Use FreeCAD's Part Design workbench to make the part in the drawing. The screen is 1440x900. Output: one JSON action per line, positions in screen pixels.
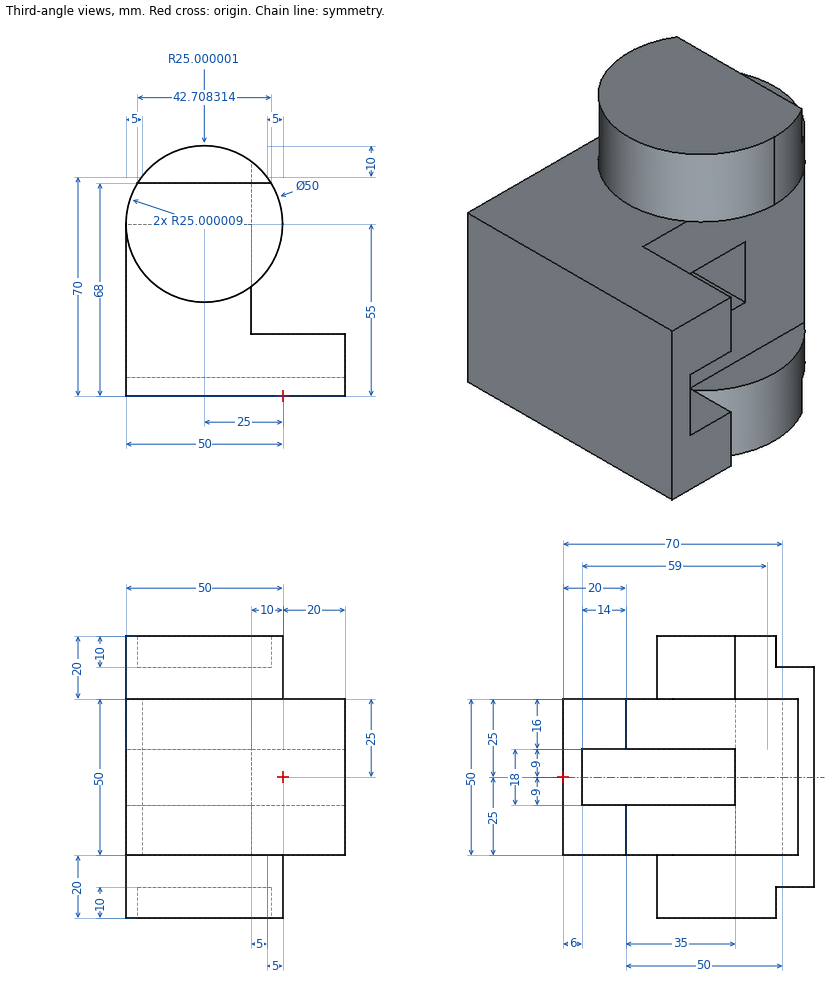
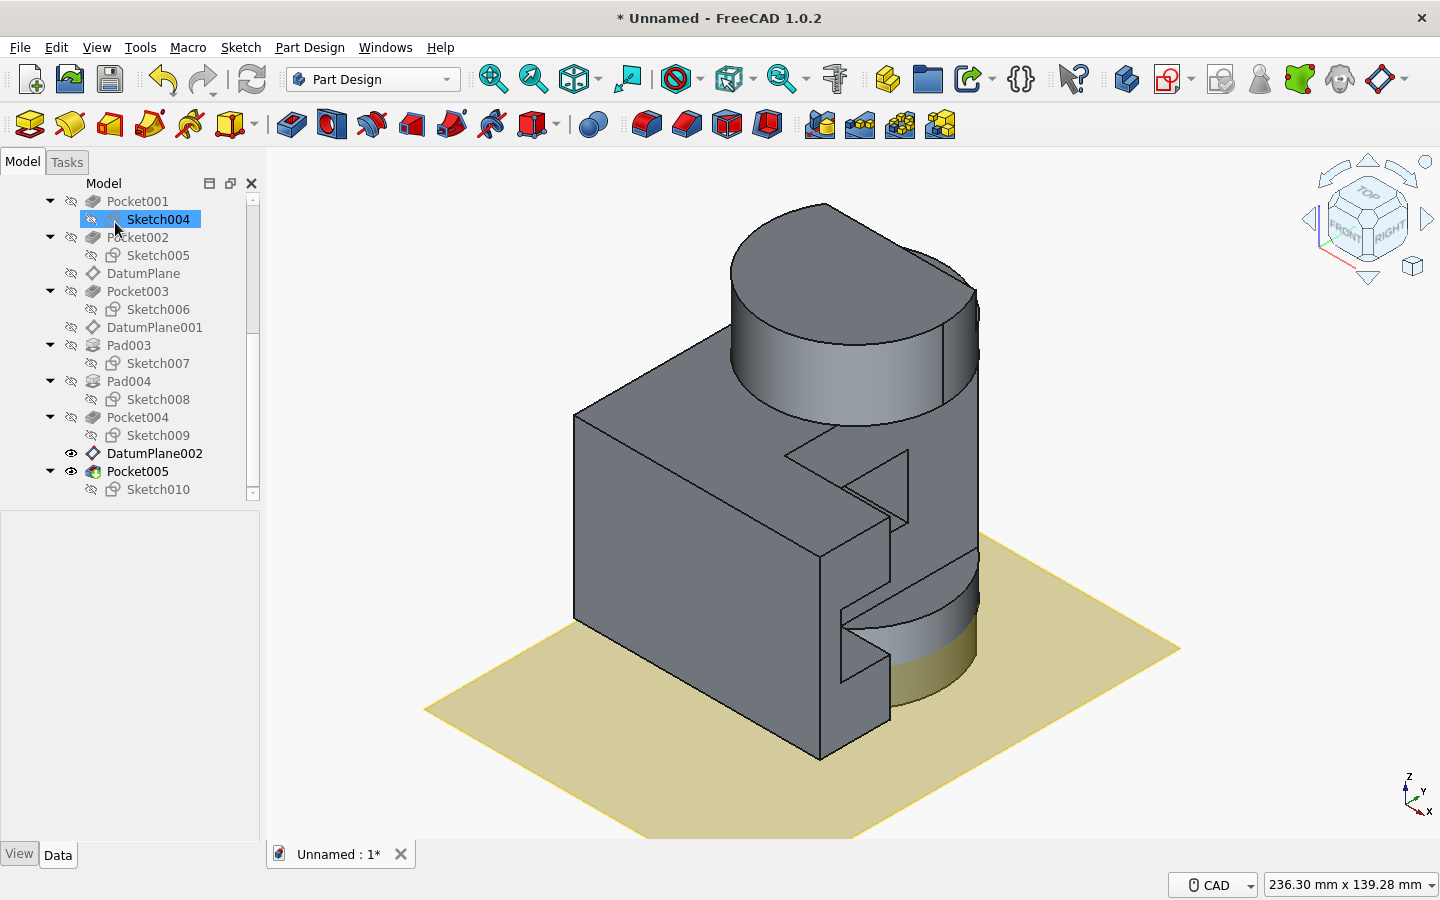
{"action": "left_click", "coordinate": [116, 453]}
{"action": "key", "text": "space"}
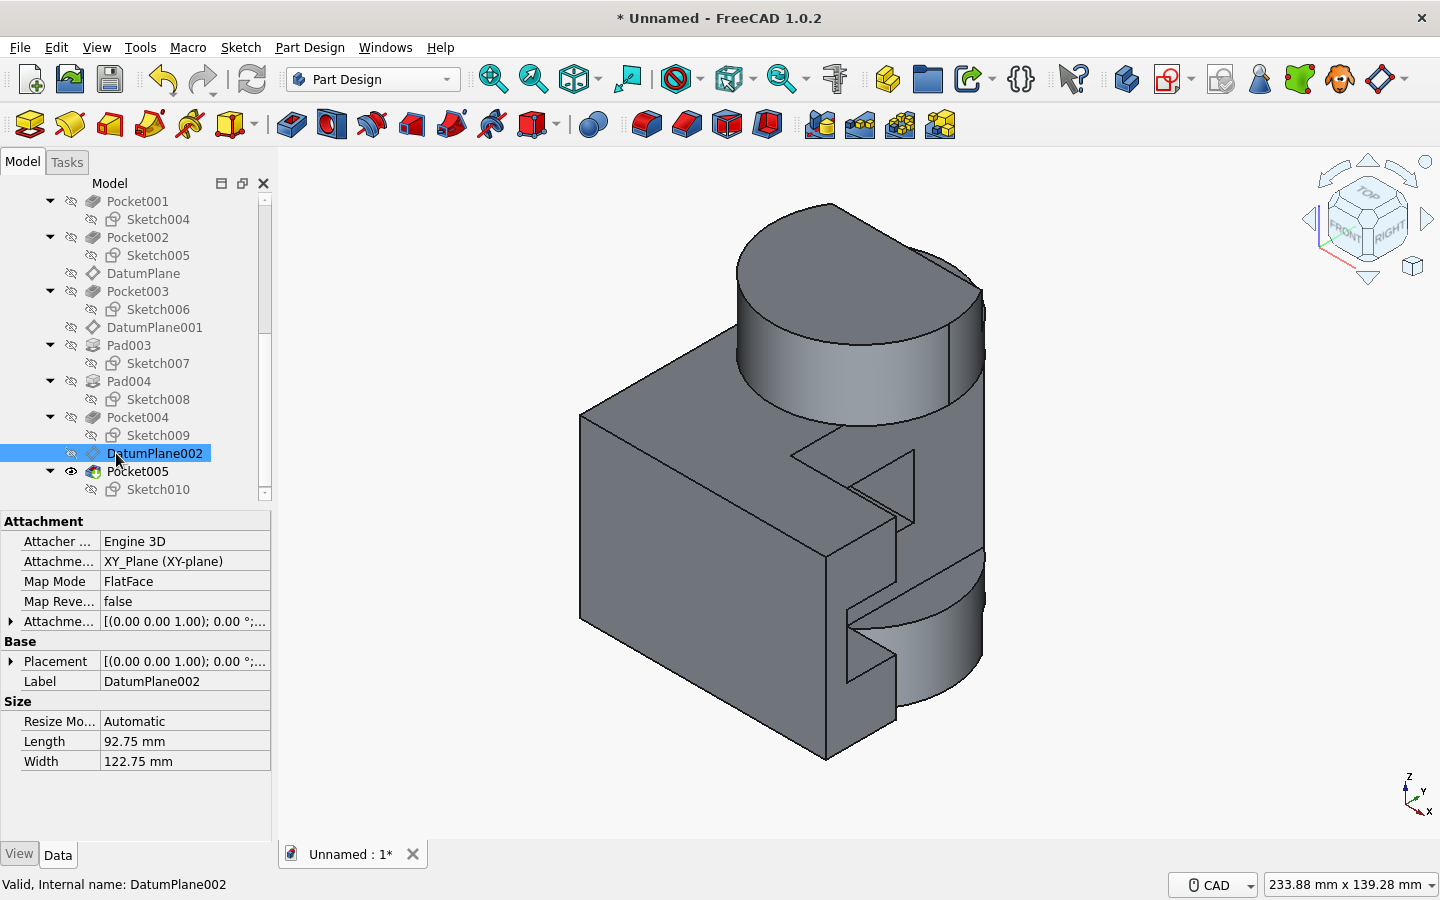
{"action": "left_click", "coordinate": [494, 80]}